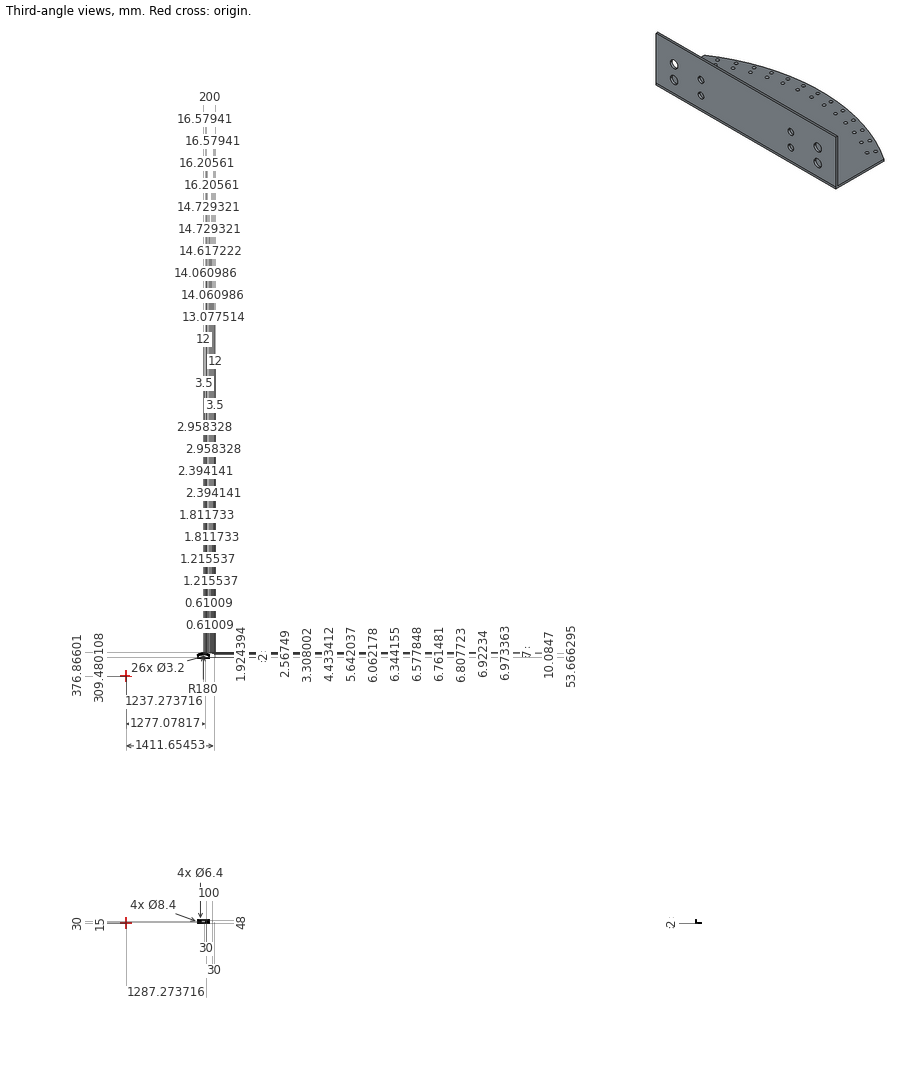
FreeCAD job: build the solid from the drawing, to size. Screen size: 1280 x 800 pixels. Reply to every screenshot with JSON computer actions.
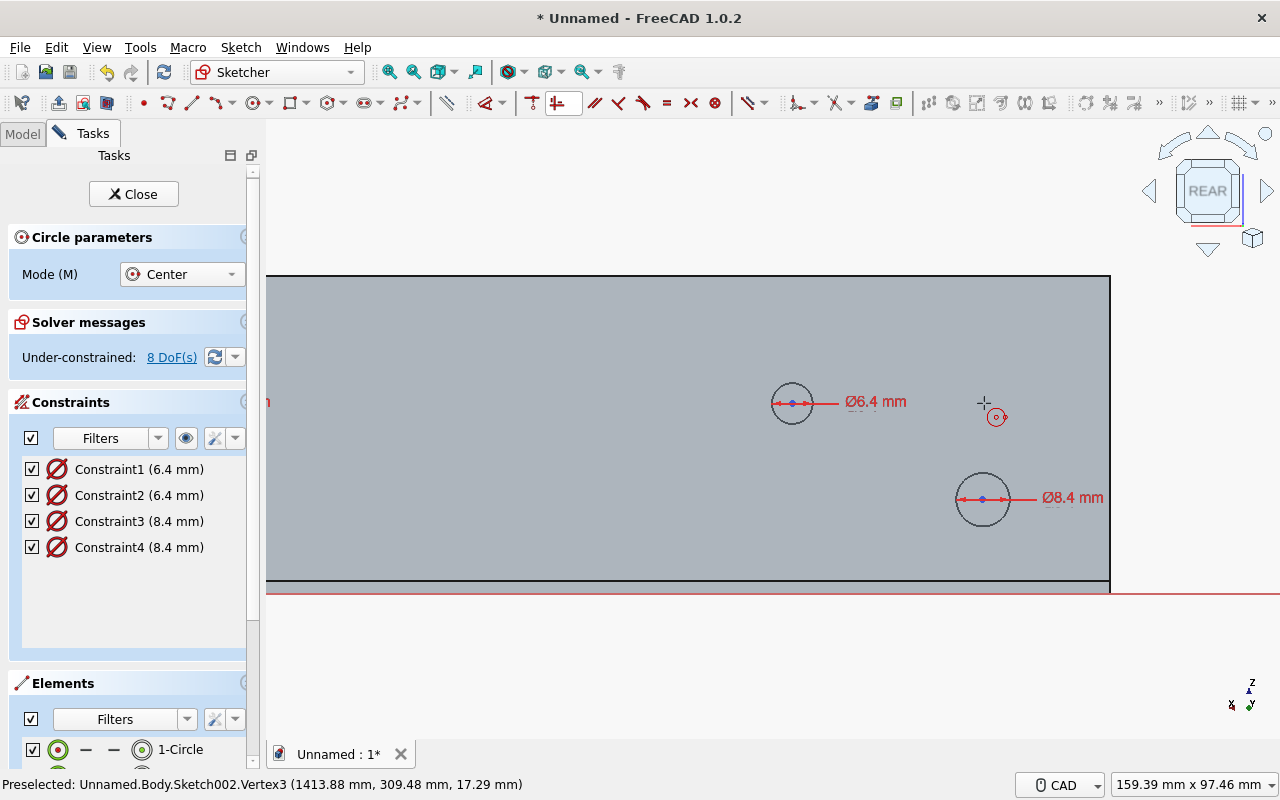
{"action": "left_click", "coordinate": [983, 403]}
{"action": "mouse_move", "coordinate": [1002, 384]}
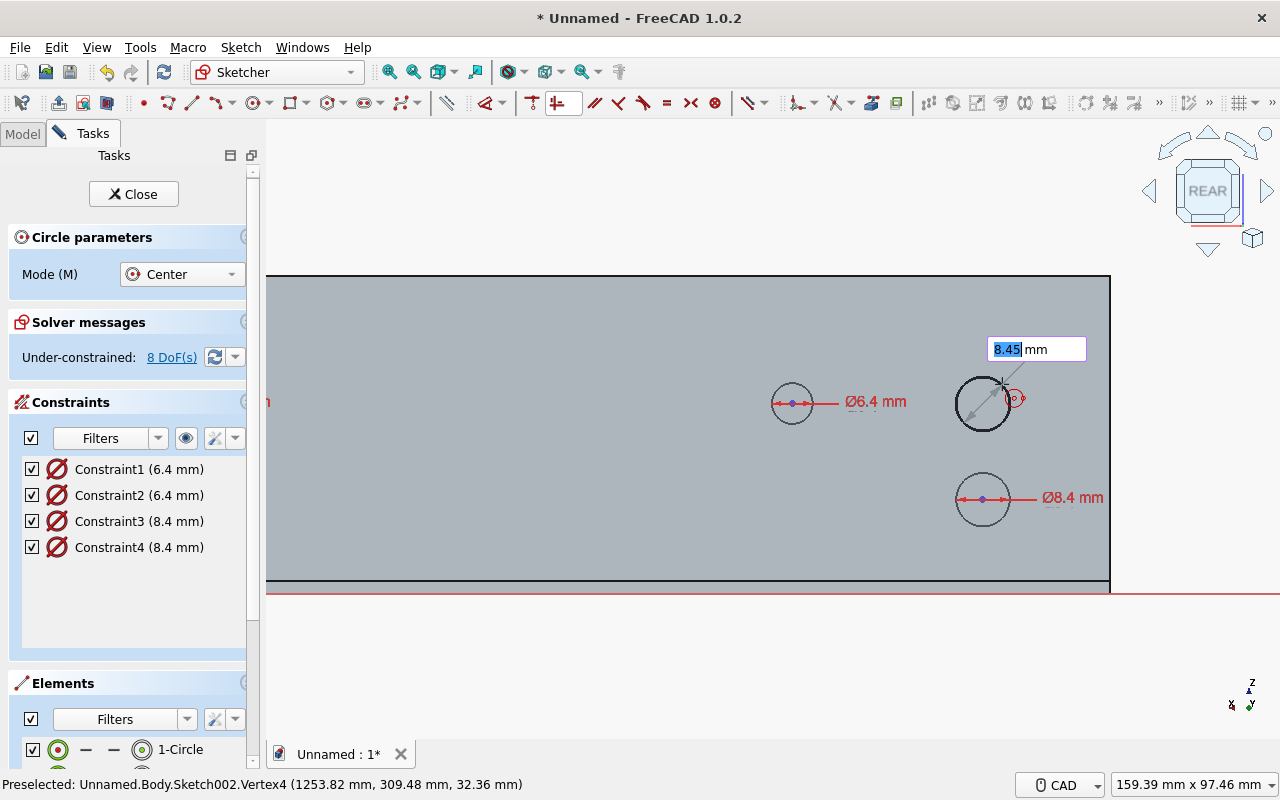
{"action": "type", "text": "8.4"}
{"action": "key", "text": "Return"}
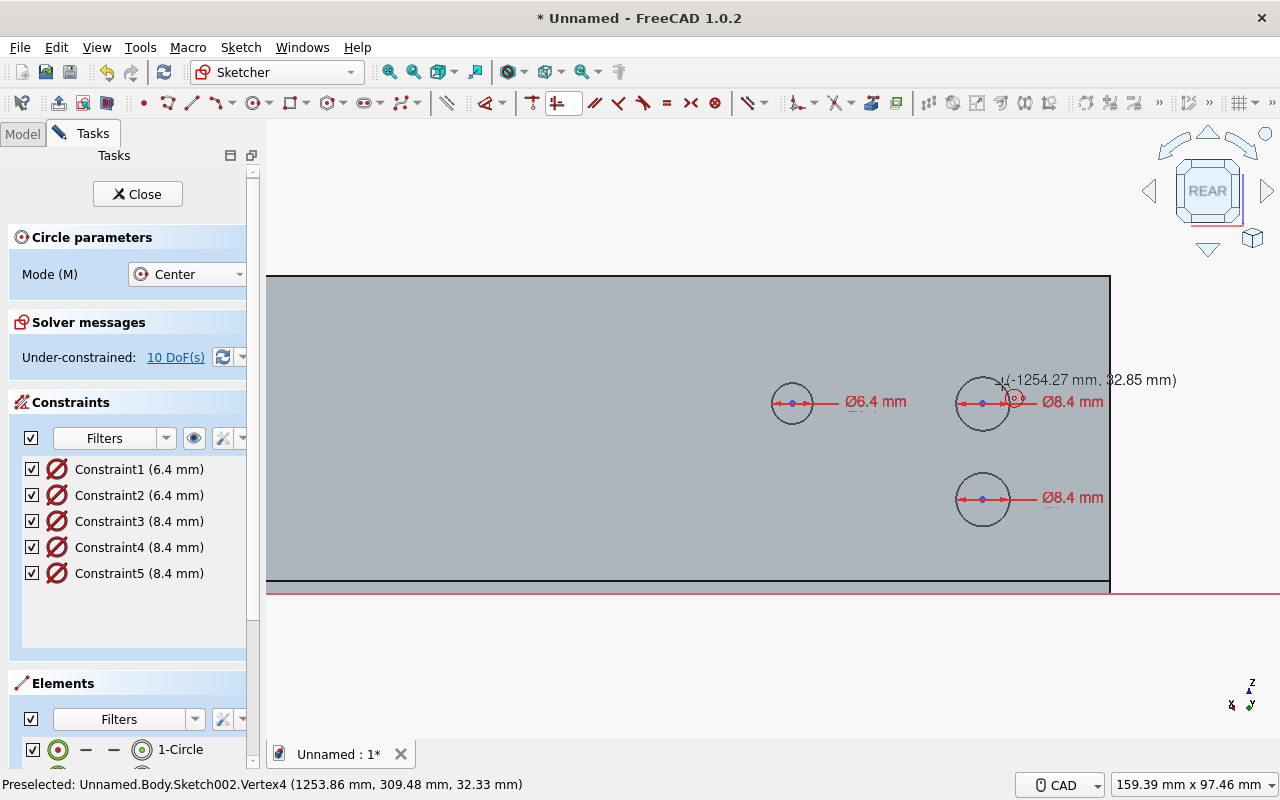
{"action": "left_click", "coordinate": [792, 499]}
{"action": "mouse_move", "coordinate": [806, 484]}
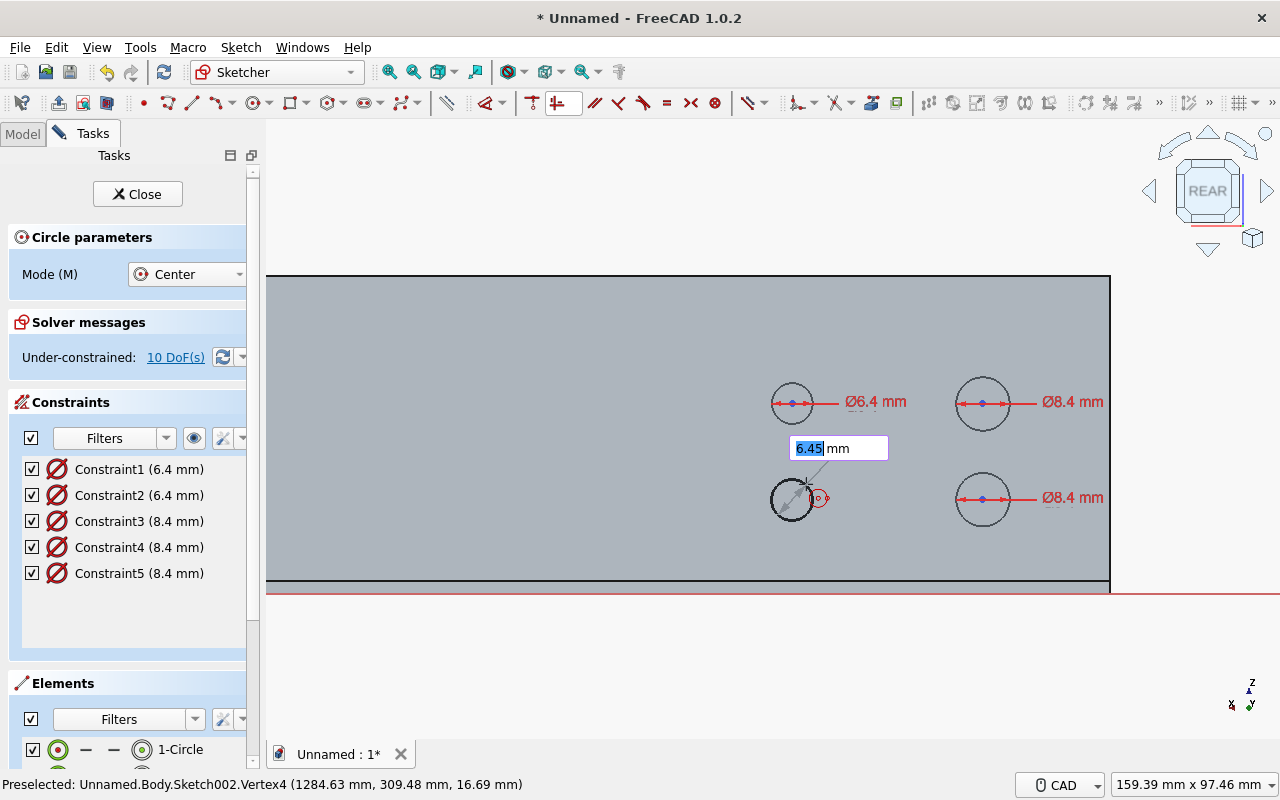
{"action": "type", "text": "6.4"}
{"action": "key", "text": "Return"}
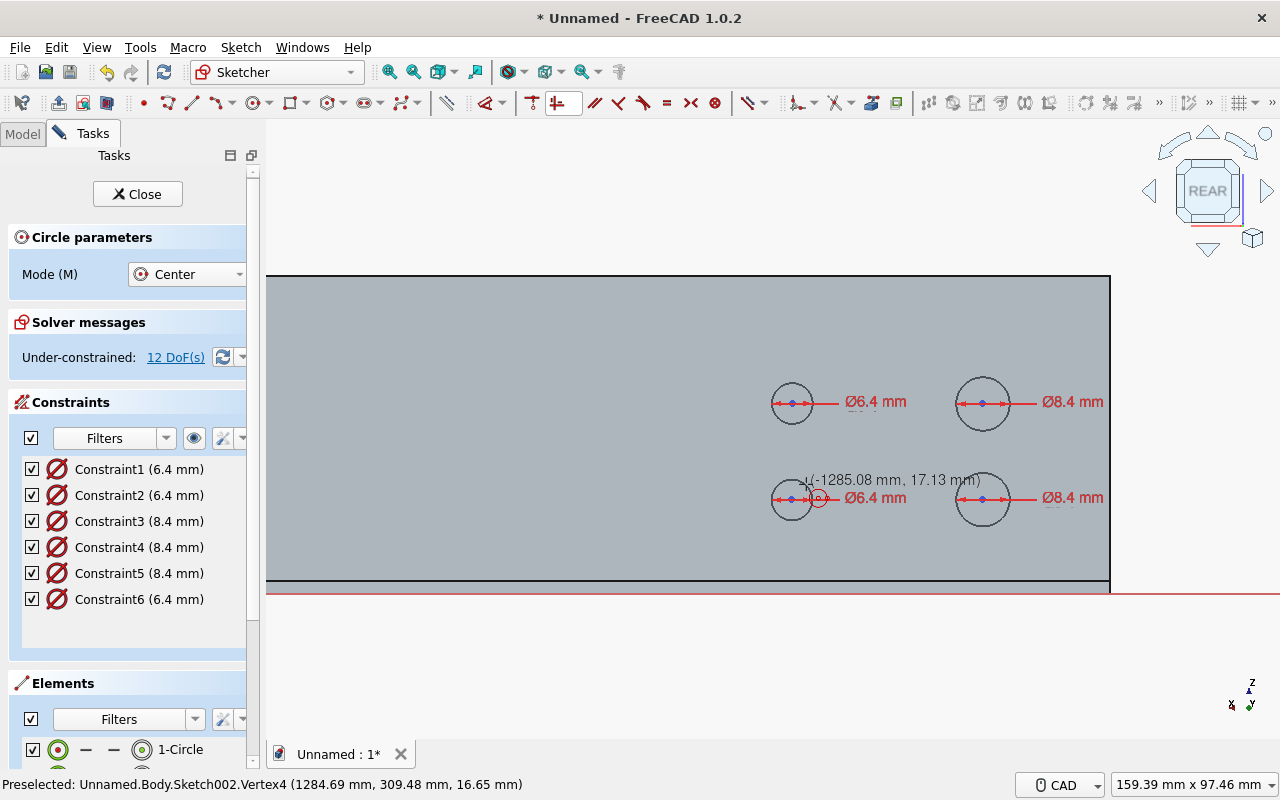
{"action": "scroll", "coordinate": [985, 402], "scroll_direction": "down", "scroll_amount": 3}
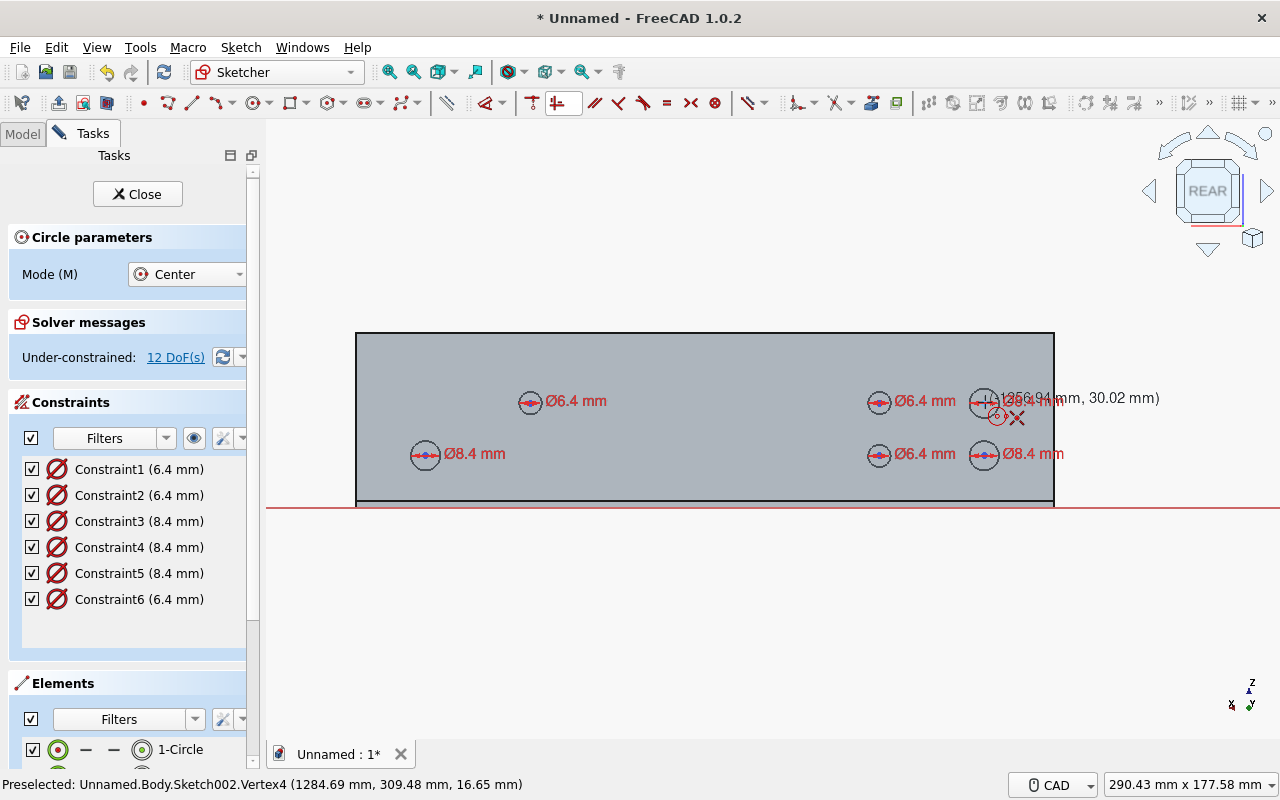
{"action": "scroll", "coordinate": [530, 455], "scroll_direction": "up", "scroll_amount": 4}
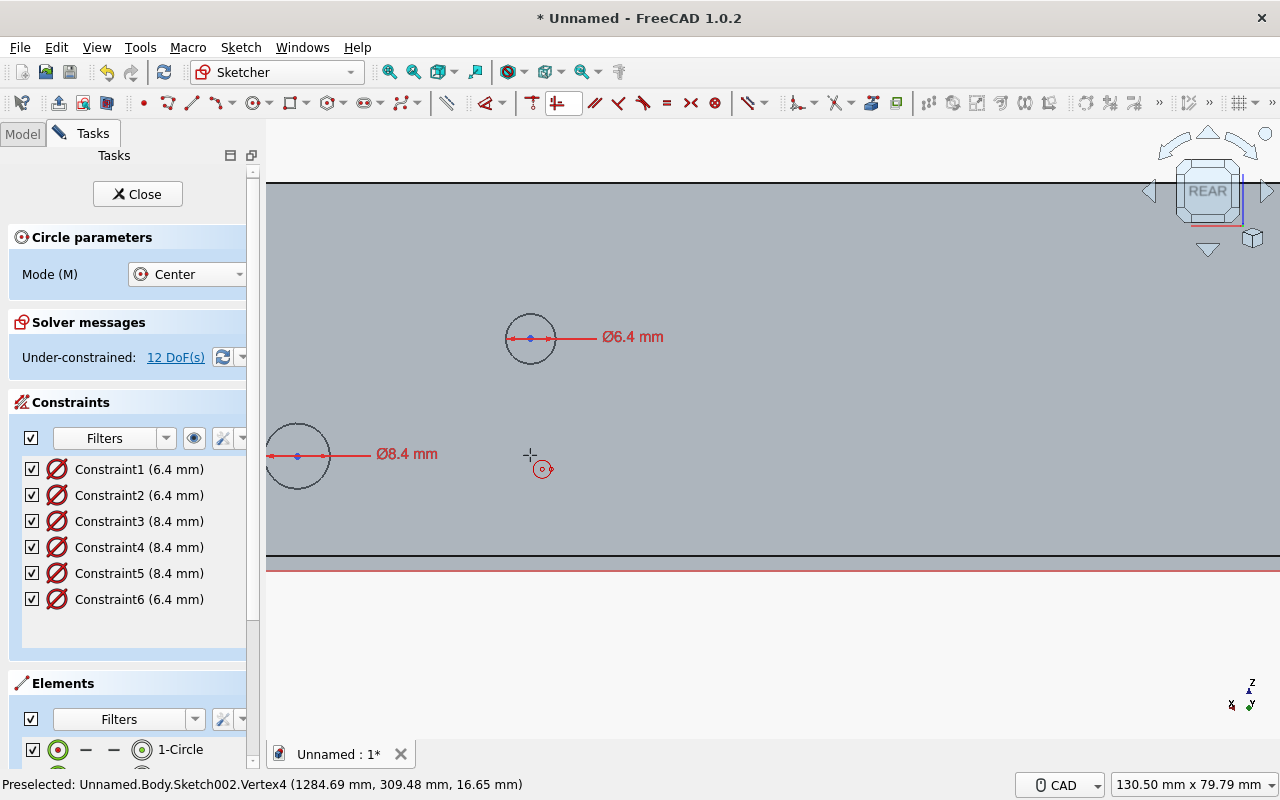
{"action": "left_click", "coordinate": [530, 455]}
{"action": "mouse_move", "coordinate": [548, 437]}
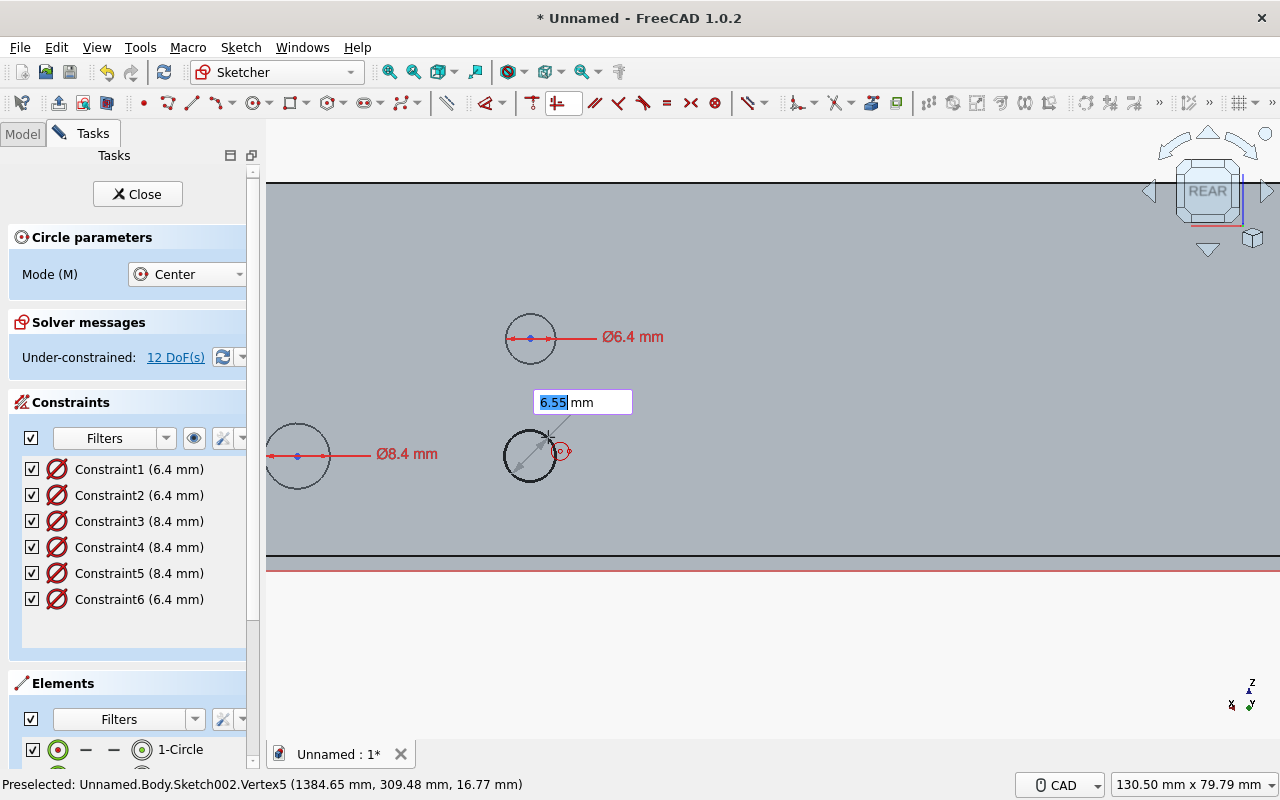
{"action": "type", "text": "6.4"}
{"action": "key", "text": "Return"}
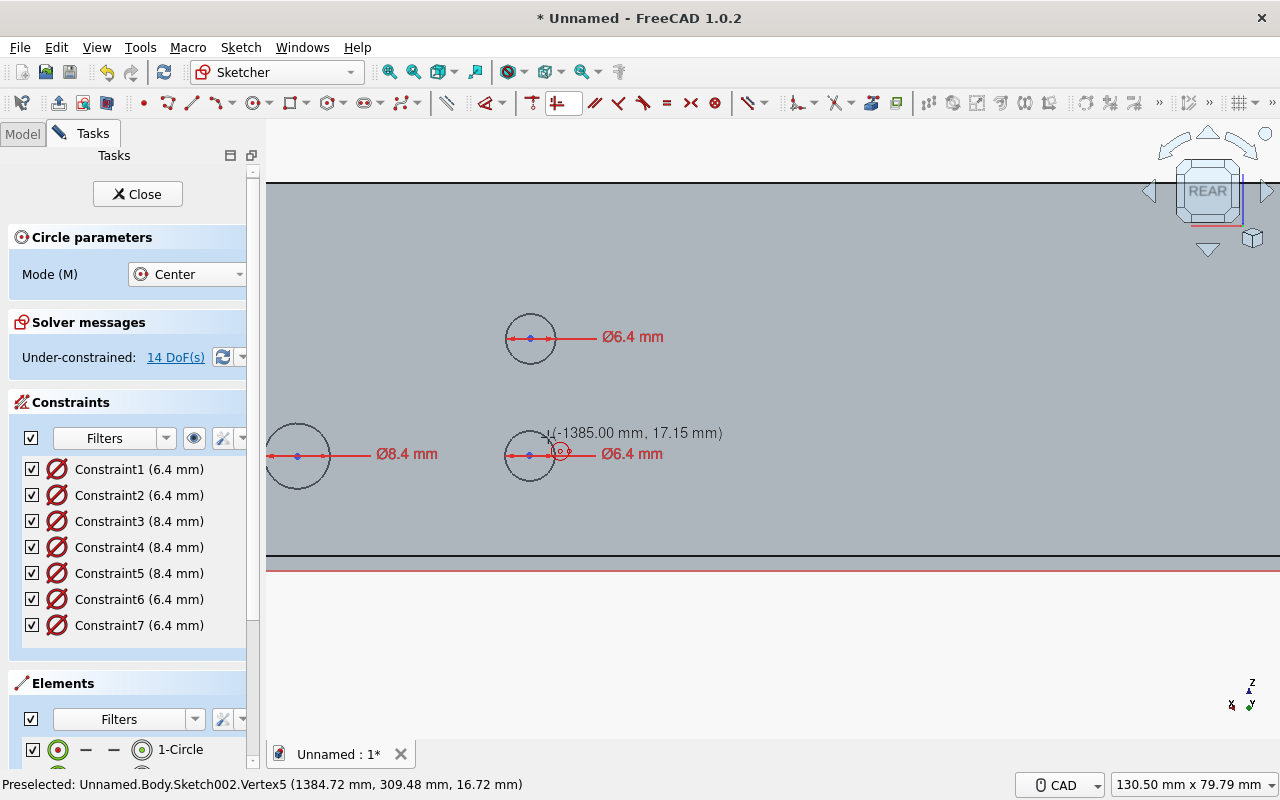
{"action": "left_click", "coordinate": [297, 338]}
{"action": "mouse_move", "coordinate": [320, 315]}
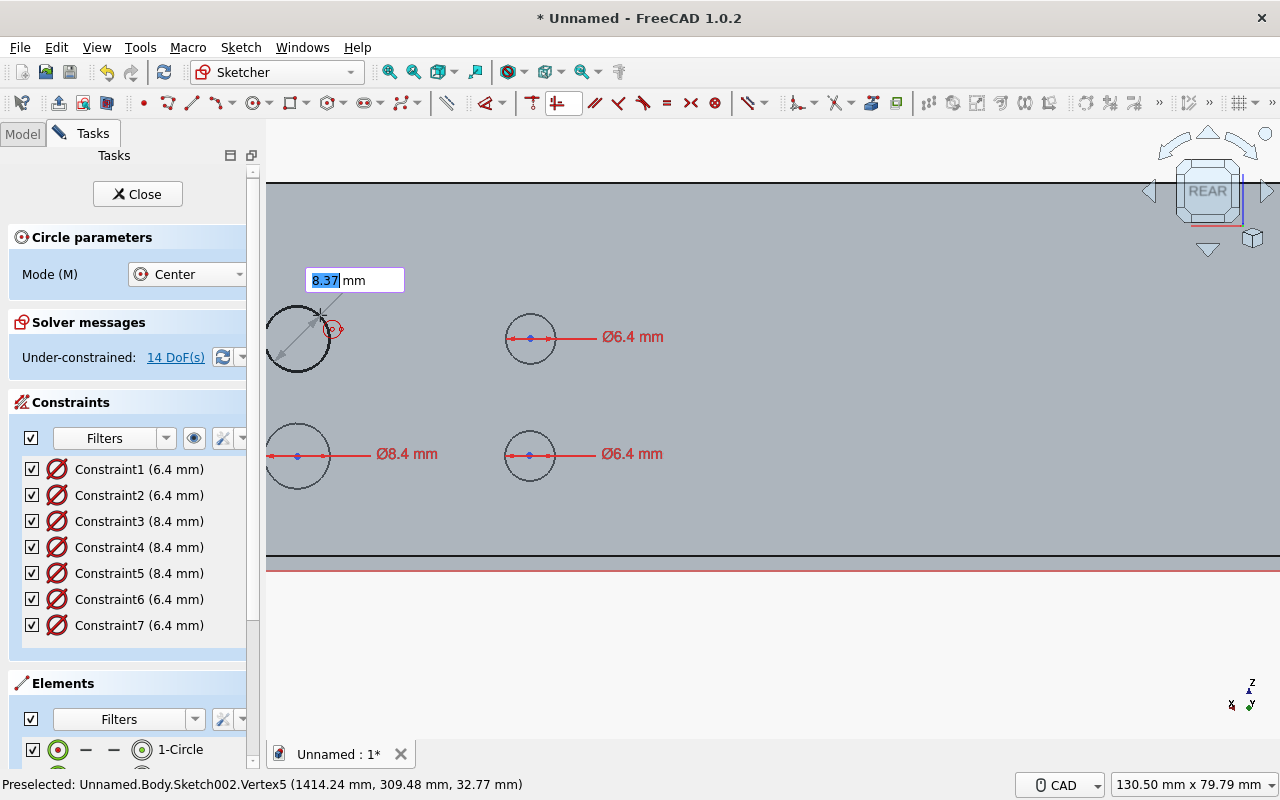
{"action": "type", "text": "8.4"}
{"action": "key", "text": "Return"}
{"action": "key", "text": "Escape"}